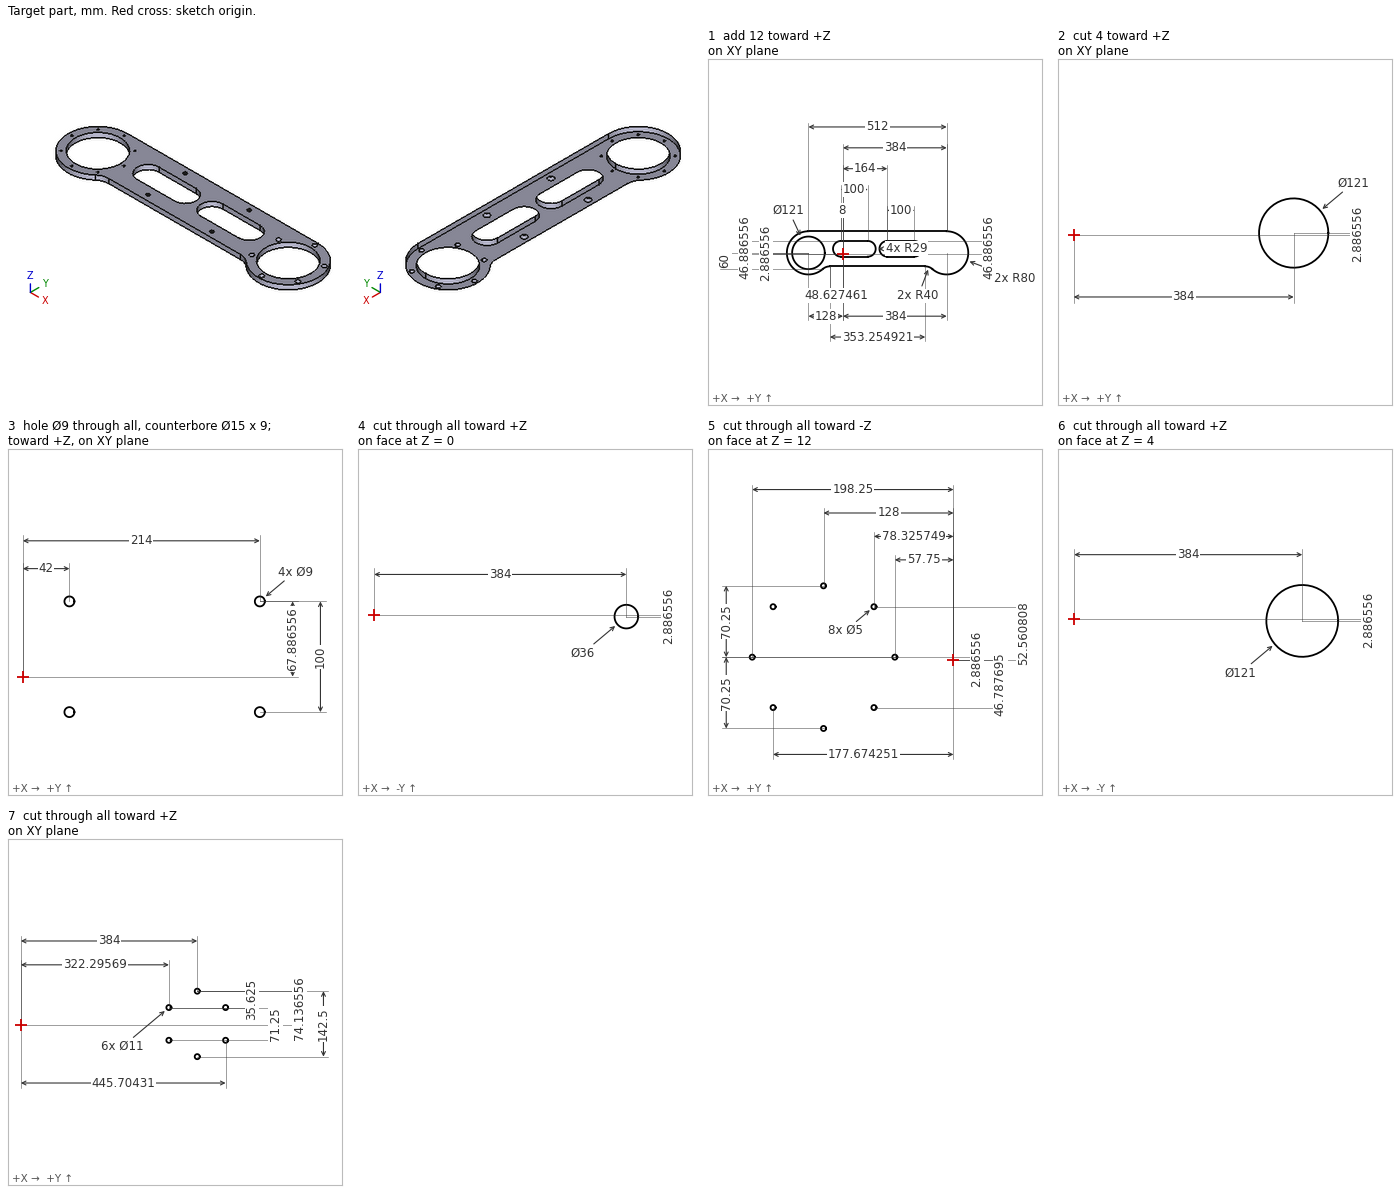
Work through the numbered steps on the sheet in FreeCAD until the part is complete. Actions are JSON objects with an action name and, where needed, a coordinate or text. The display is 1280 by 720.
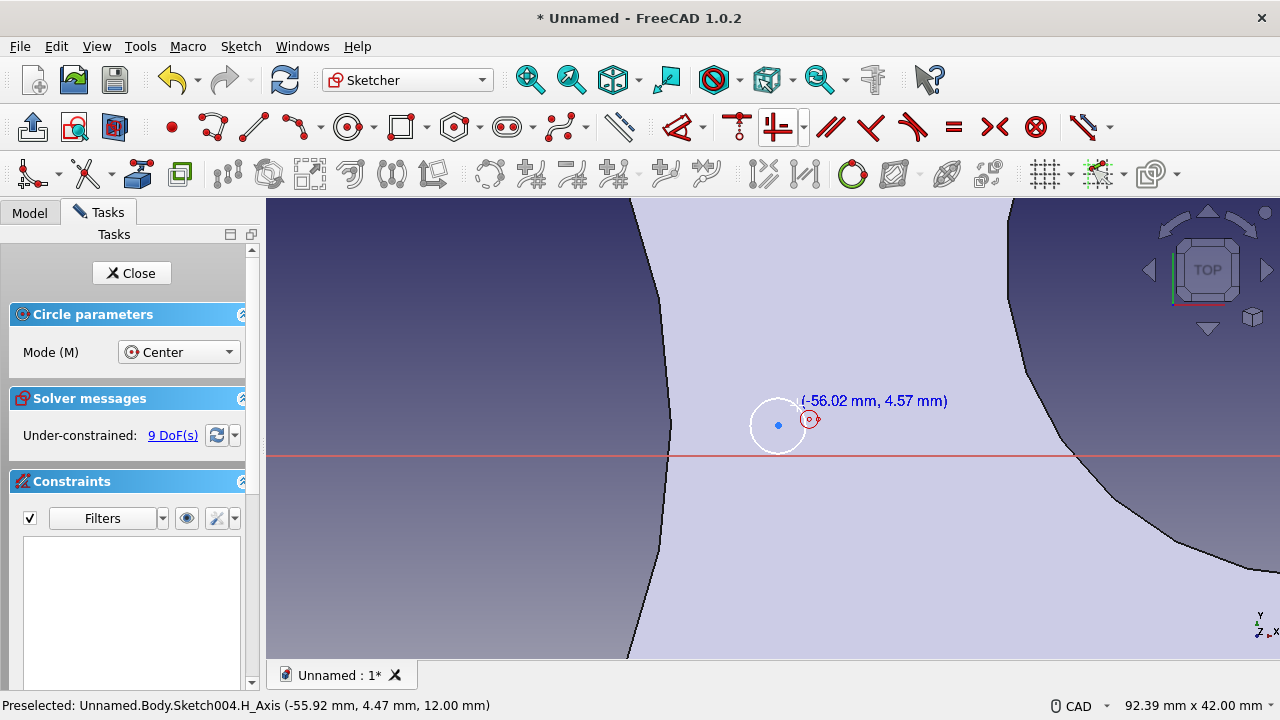
{"action": "scroll", "coordinate": [783, 429], "scroll_direction": "down", "scroll_amount": 9}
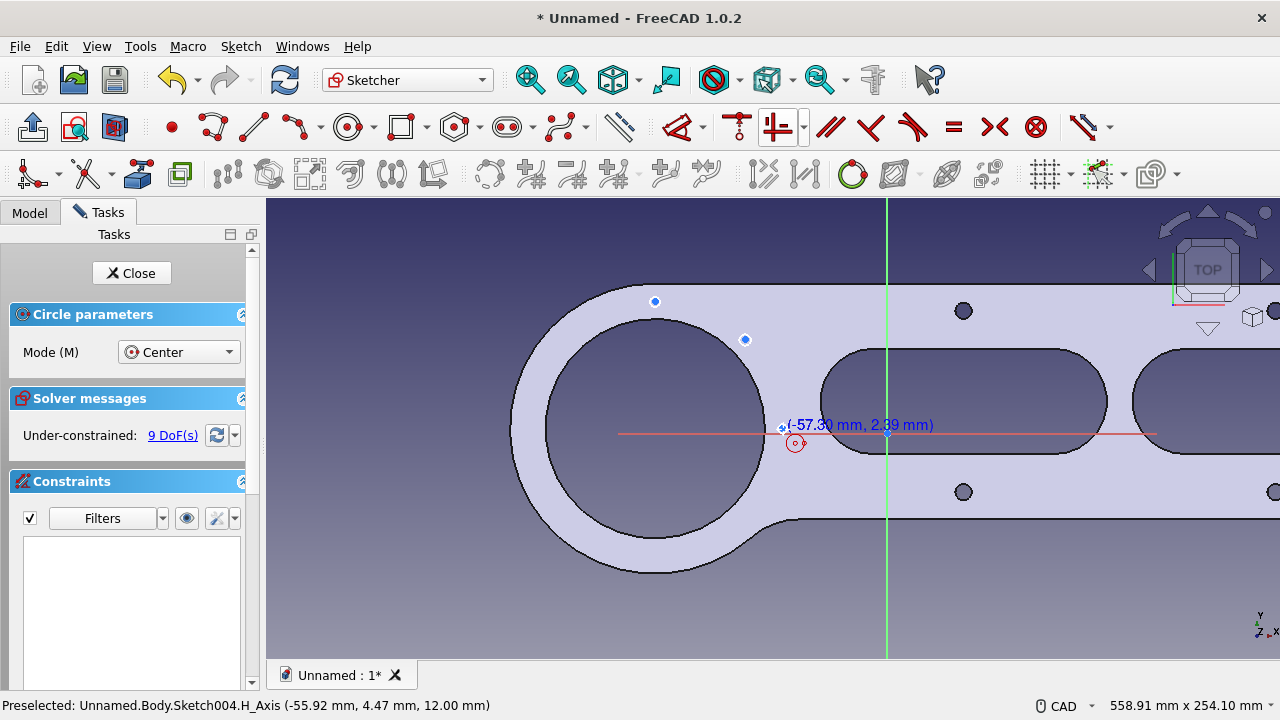
{"action": "scroll", "coordinate": [745, 519], "scroll_direction": "up", "scroll_amount": 9}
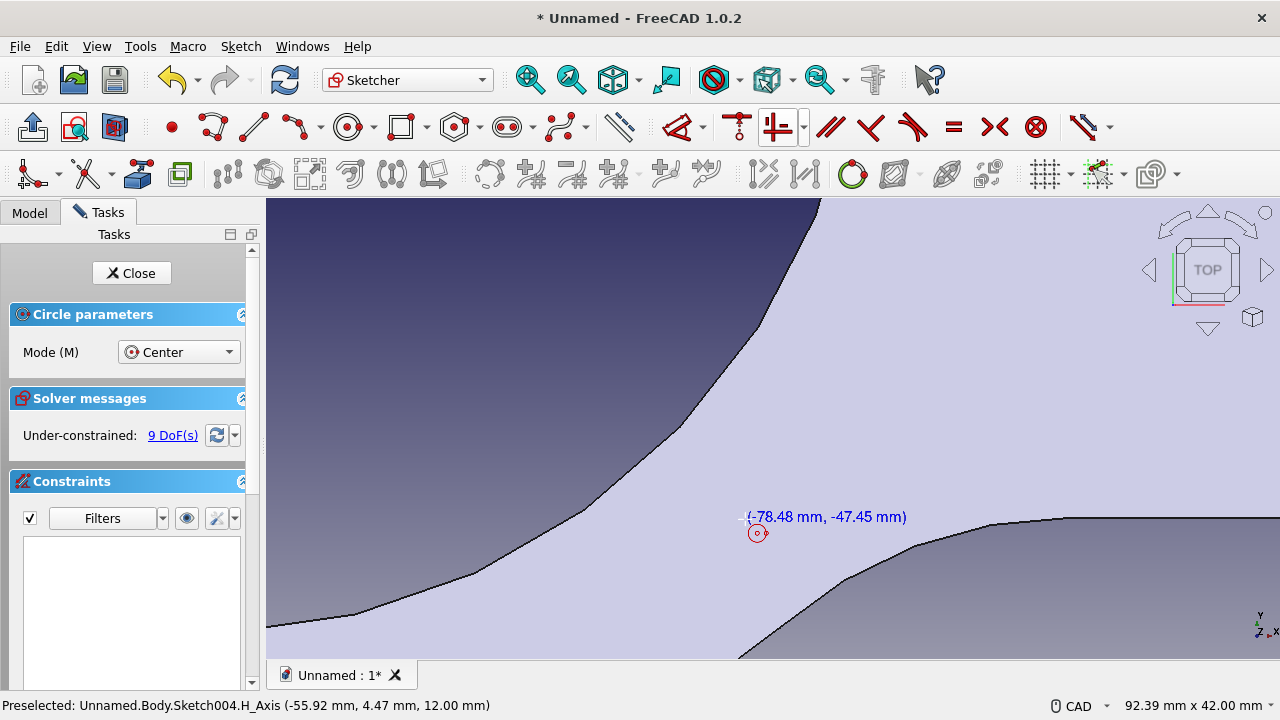
{"action": "scroll", "coordinate": [745, 519], "scroll_direction": "down", "scroll_amount": 9}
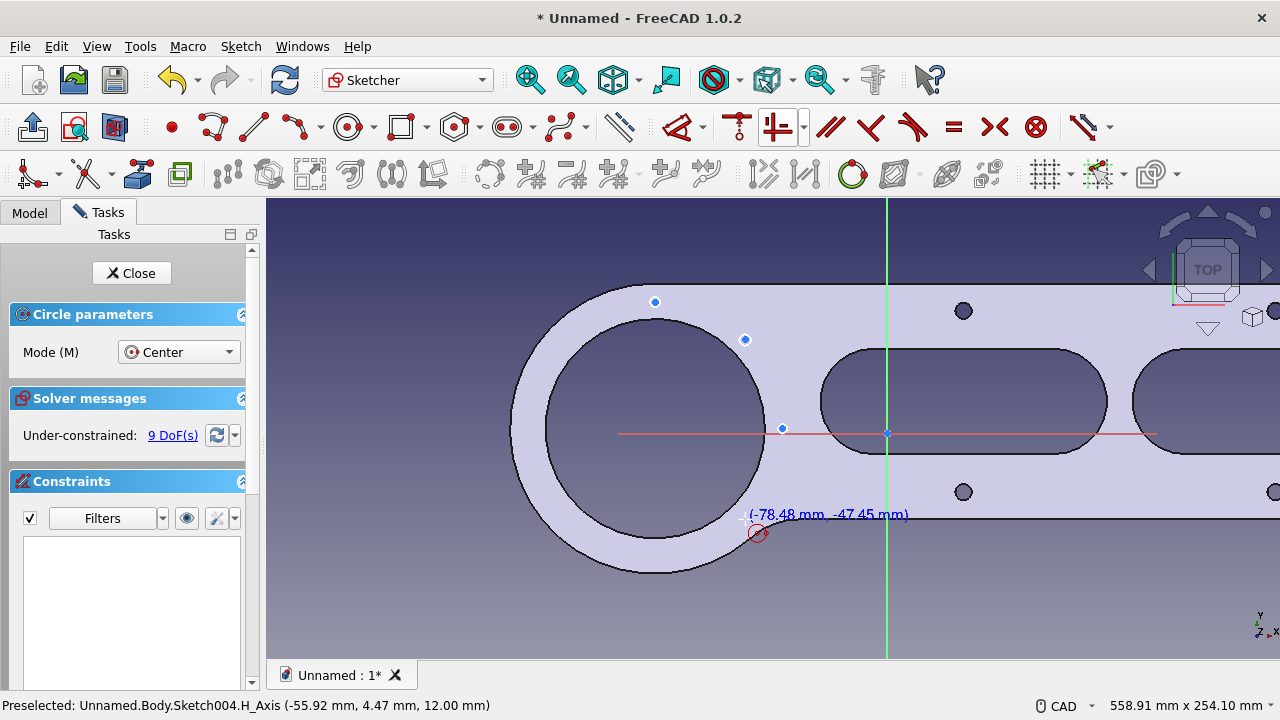
{"action": "left_click", "coordinate": [745, 519]}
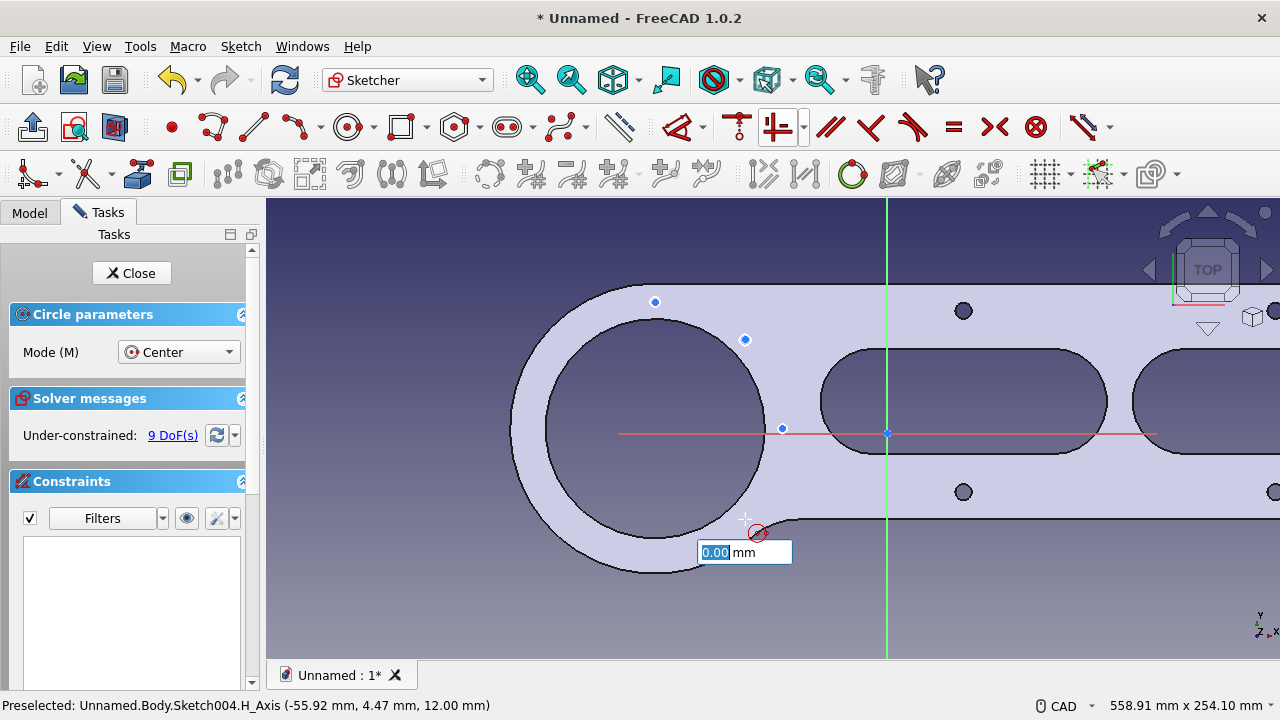
{"action": "scroll", "coordinate": [748, 516], "scroll_direction": "up", "scroll_amount": 7}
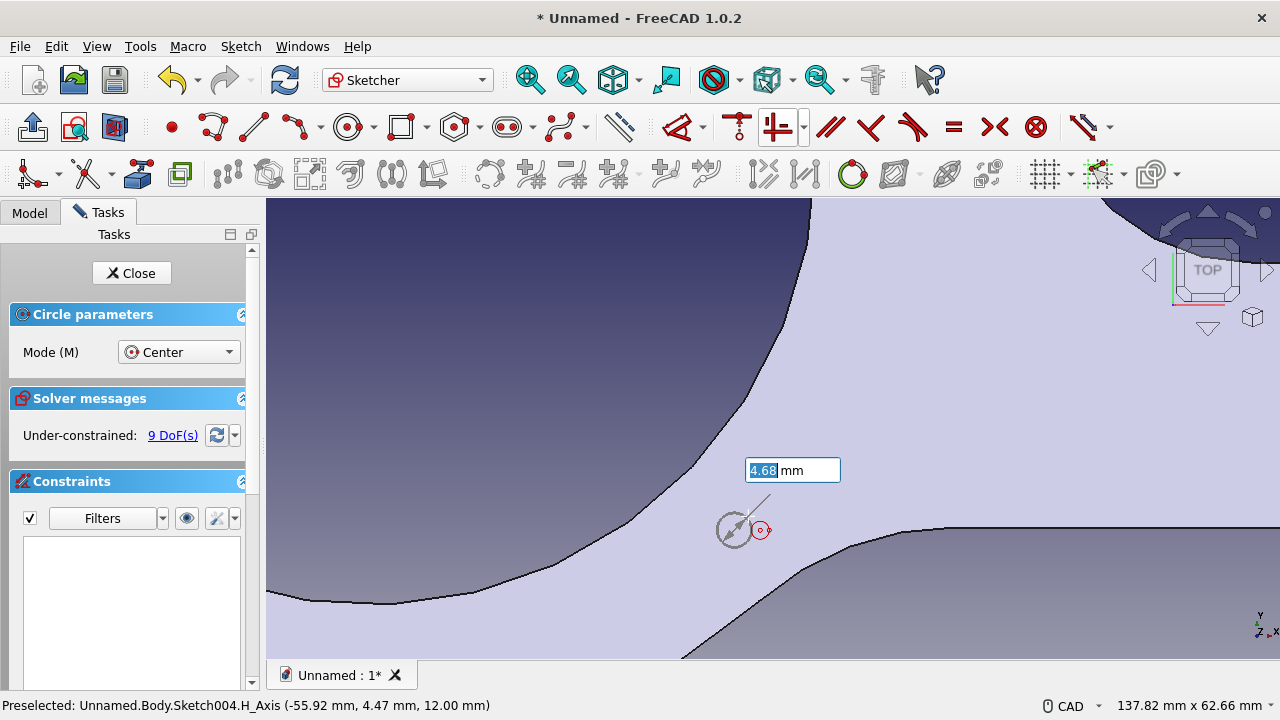
{"action": "left_click", "coordinate": [749, 512]}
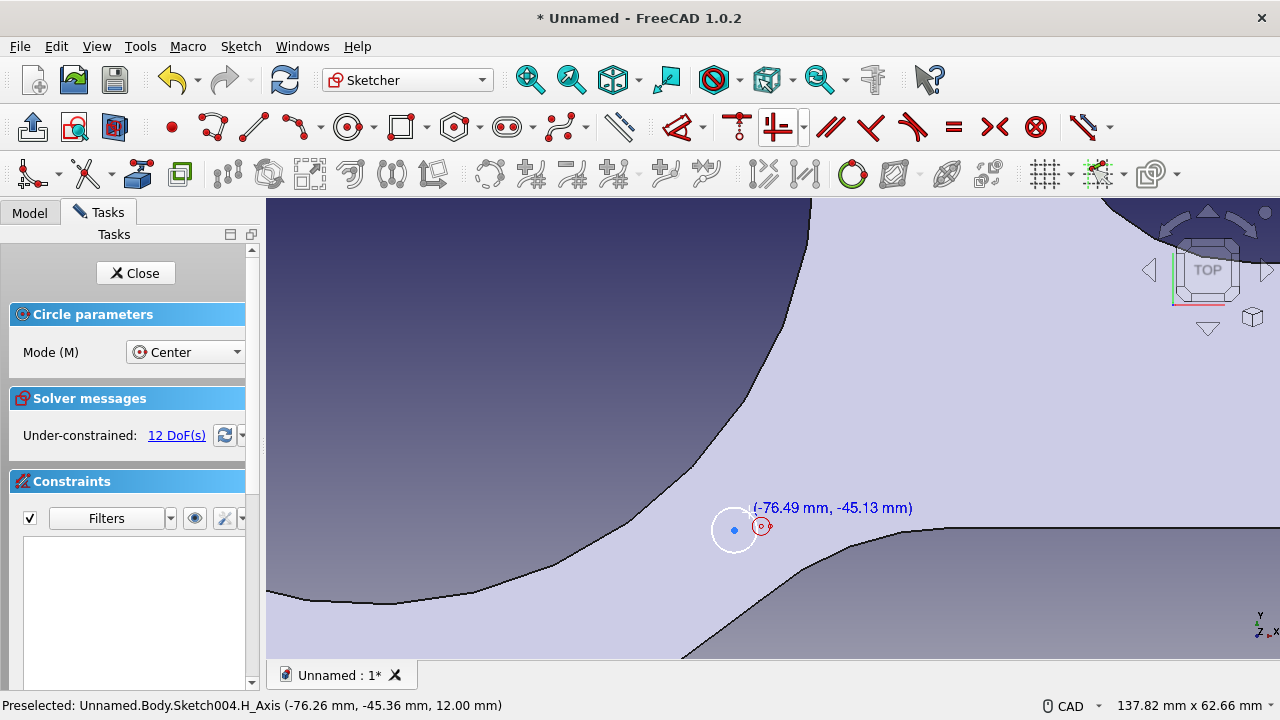
{"action": "scroll", "coordinate": [747, 516], "scroll_direction": "down", "scroll_amount": 7}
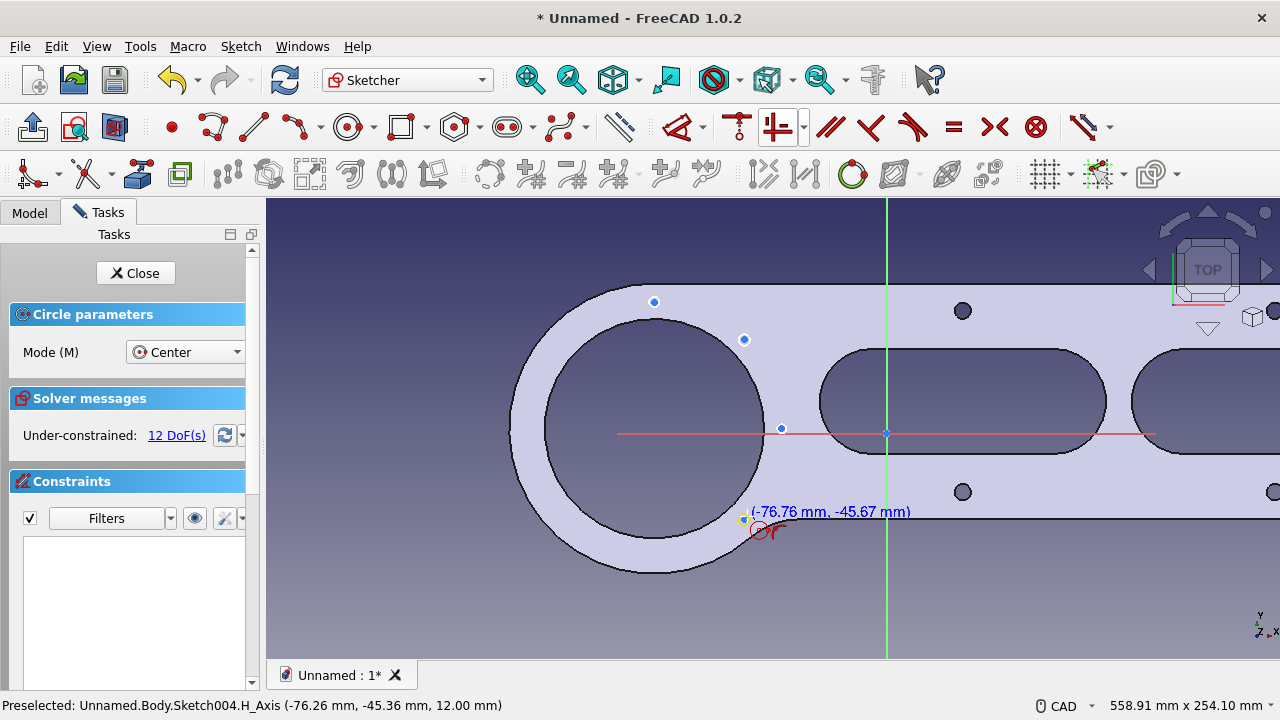
{"action": "scroll", "coordinate": [654, 556], "scroll_direction": "up", "scroll_amount": 9}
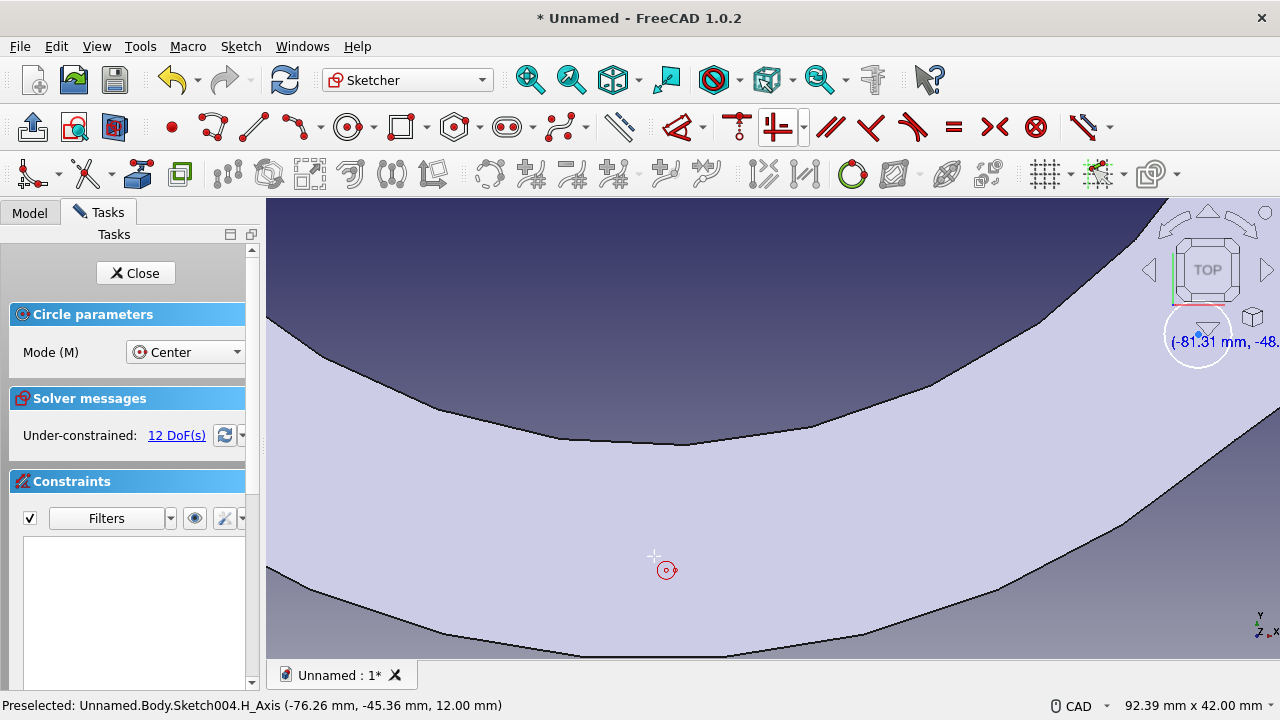
{"action": "scroll", "coordinate": [654, 557], "scroll_direction": "down", "scroll_amount": 9}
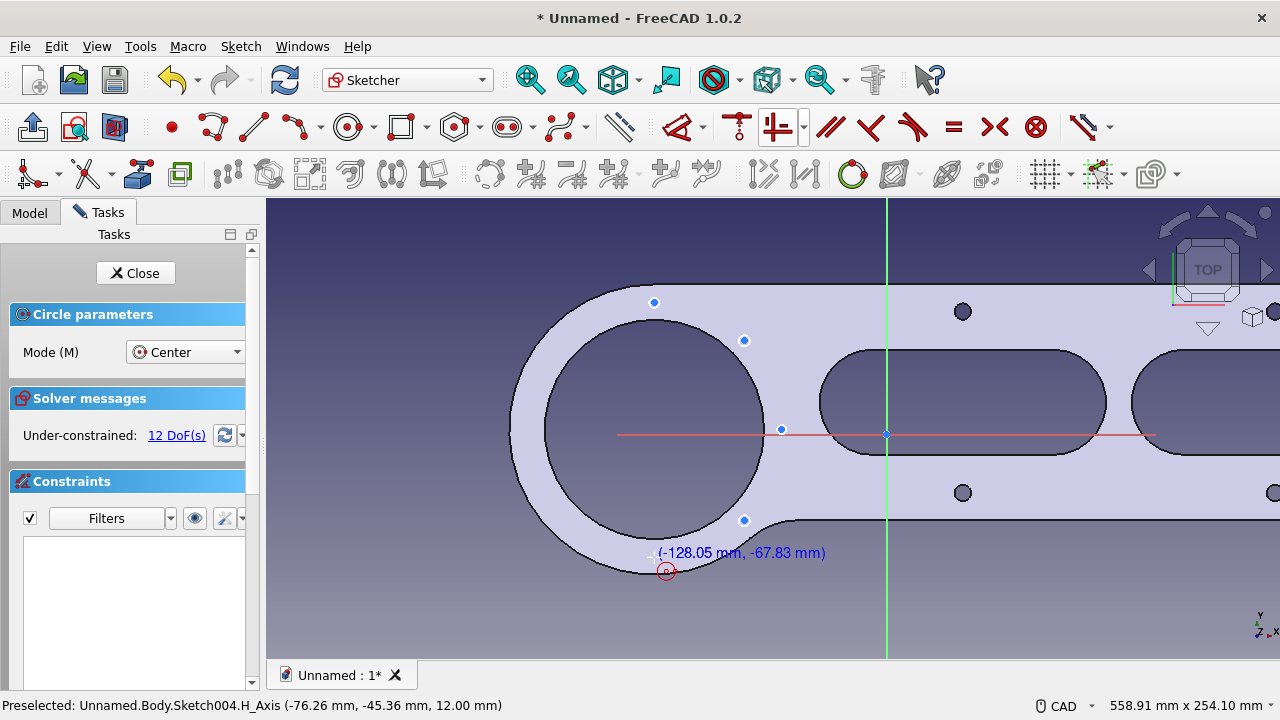
{"action": "left_click", "coordinate": [654, 557]}